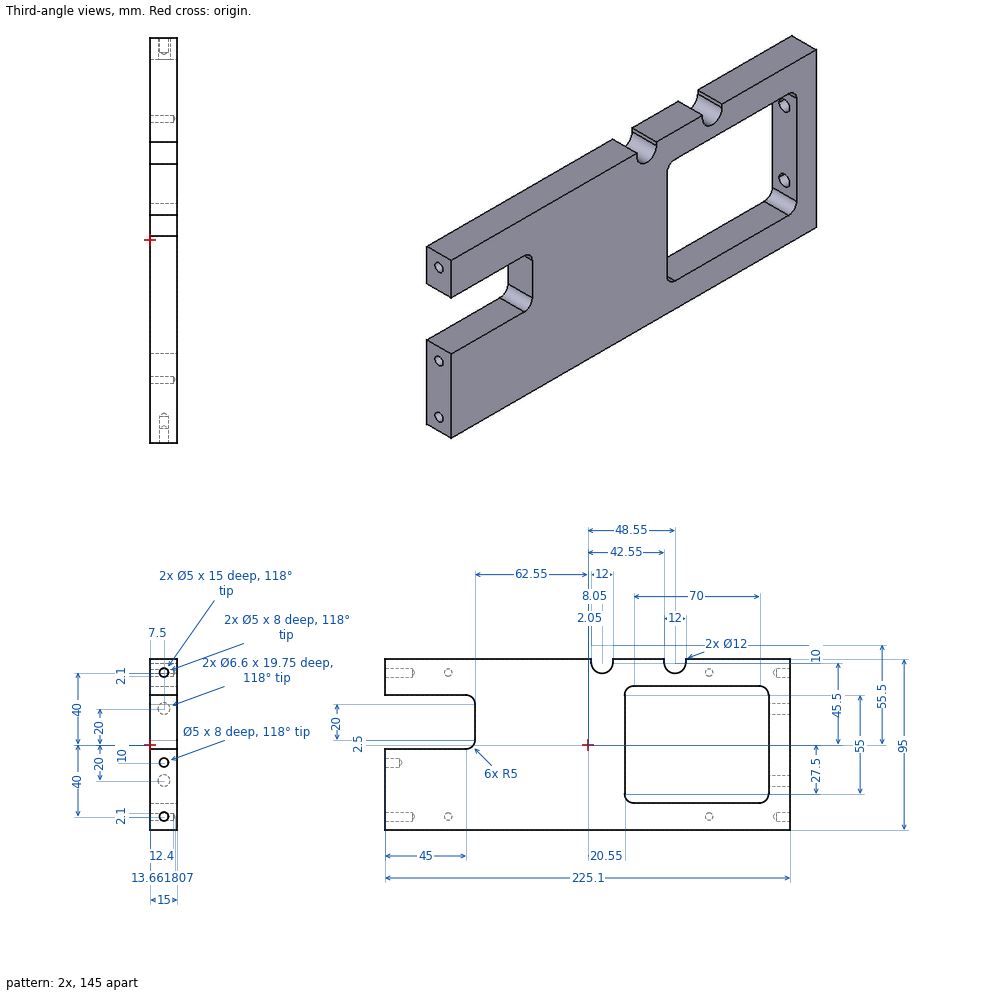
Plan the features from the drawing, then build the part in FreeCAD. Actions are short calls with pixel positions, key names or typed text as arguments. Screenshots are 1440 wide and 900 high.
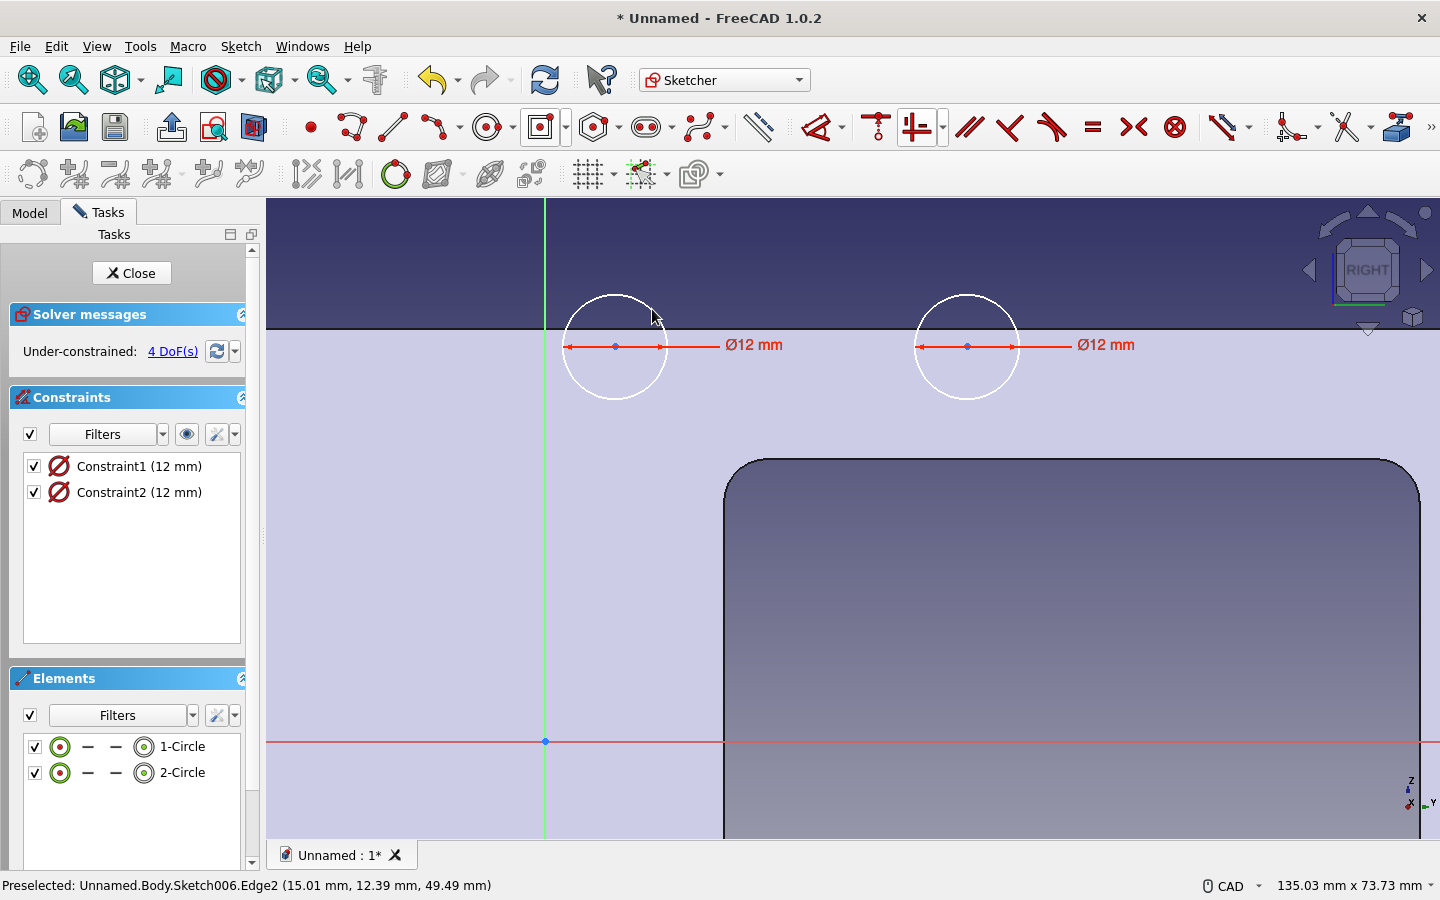
click(967, 347)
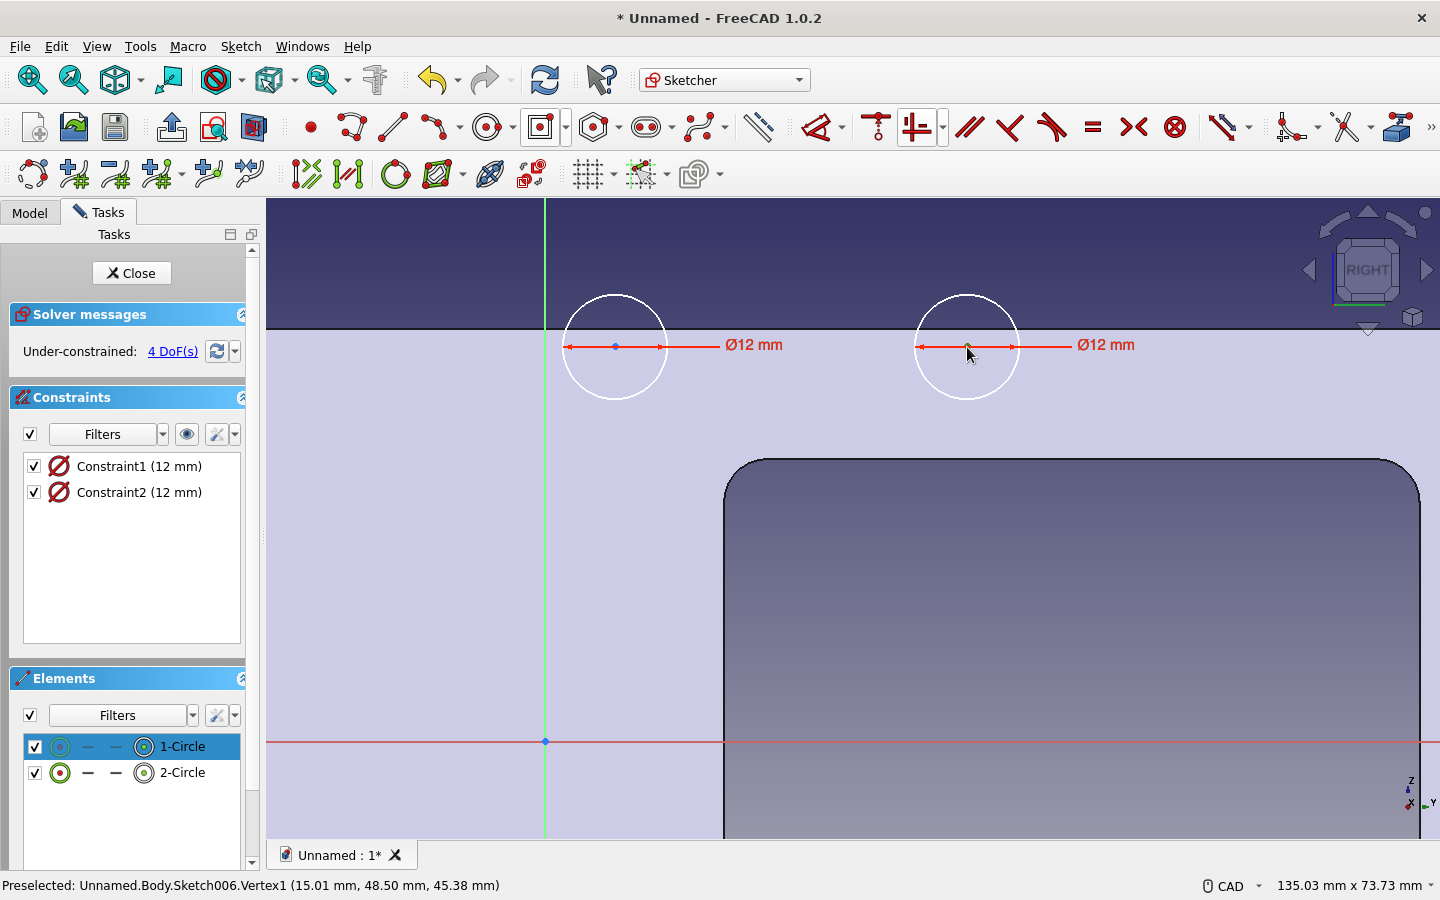
click(615, 347)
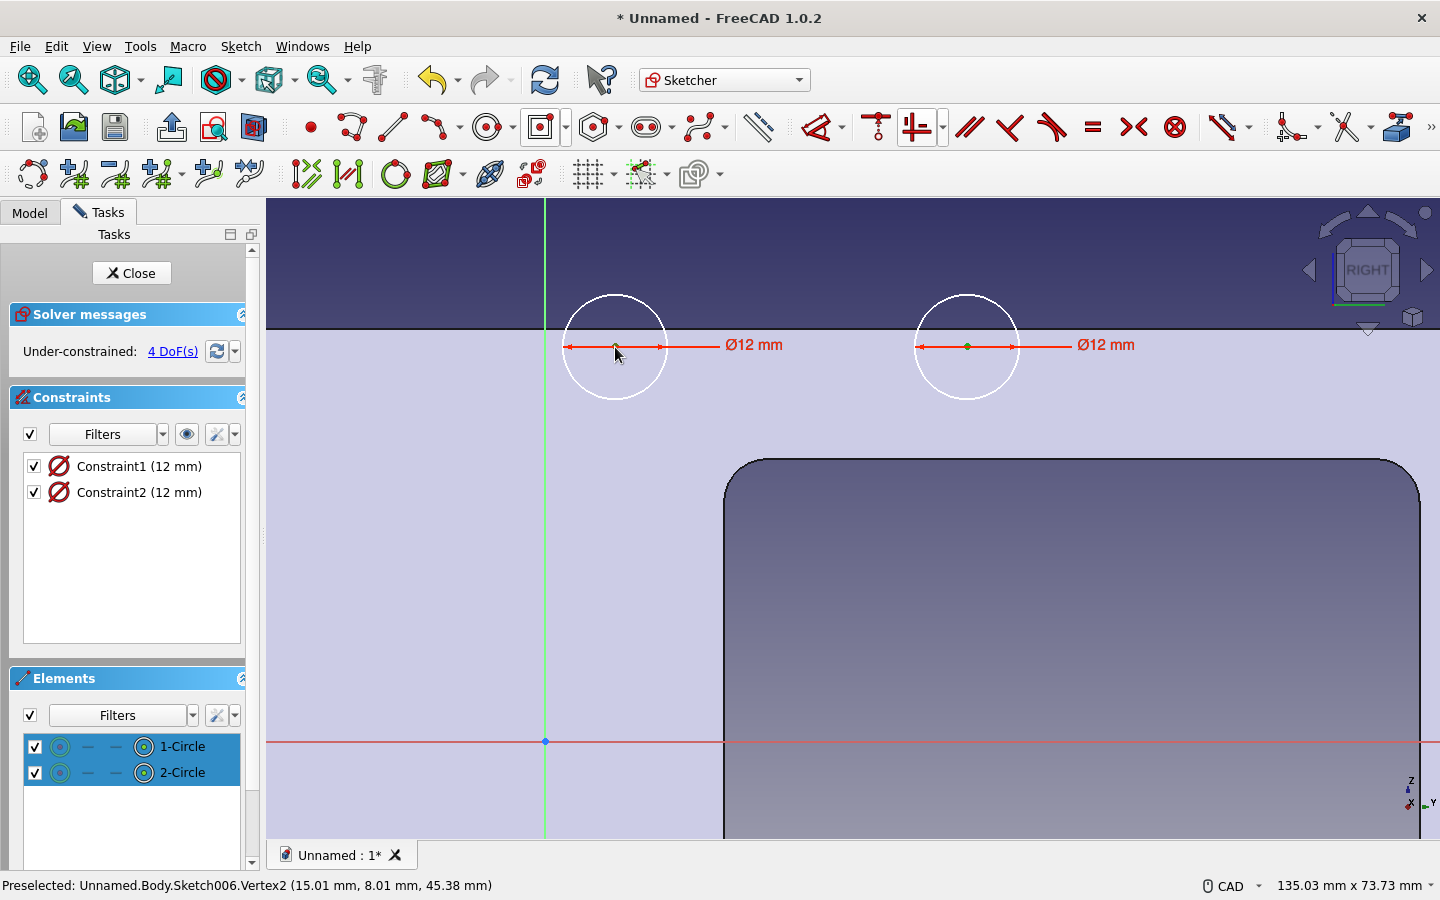
key(h)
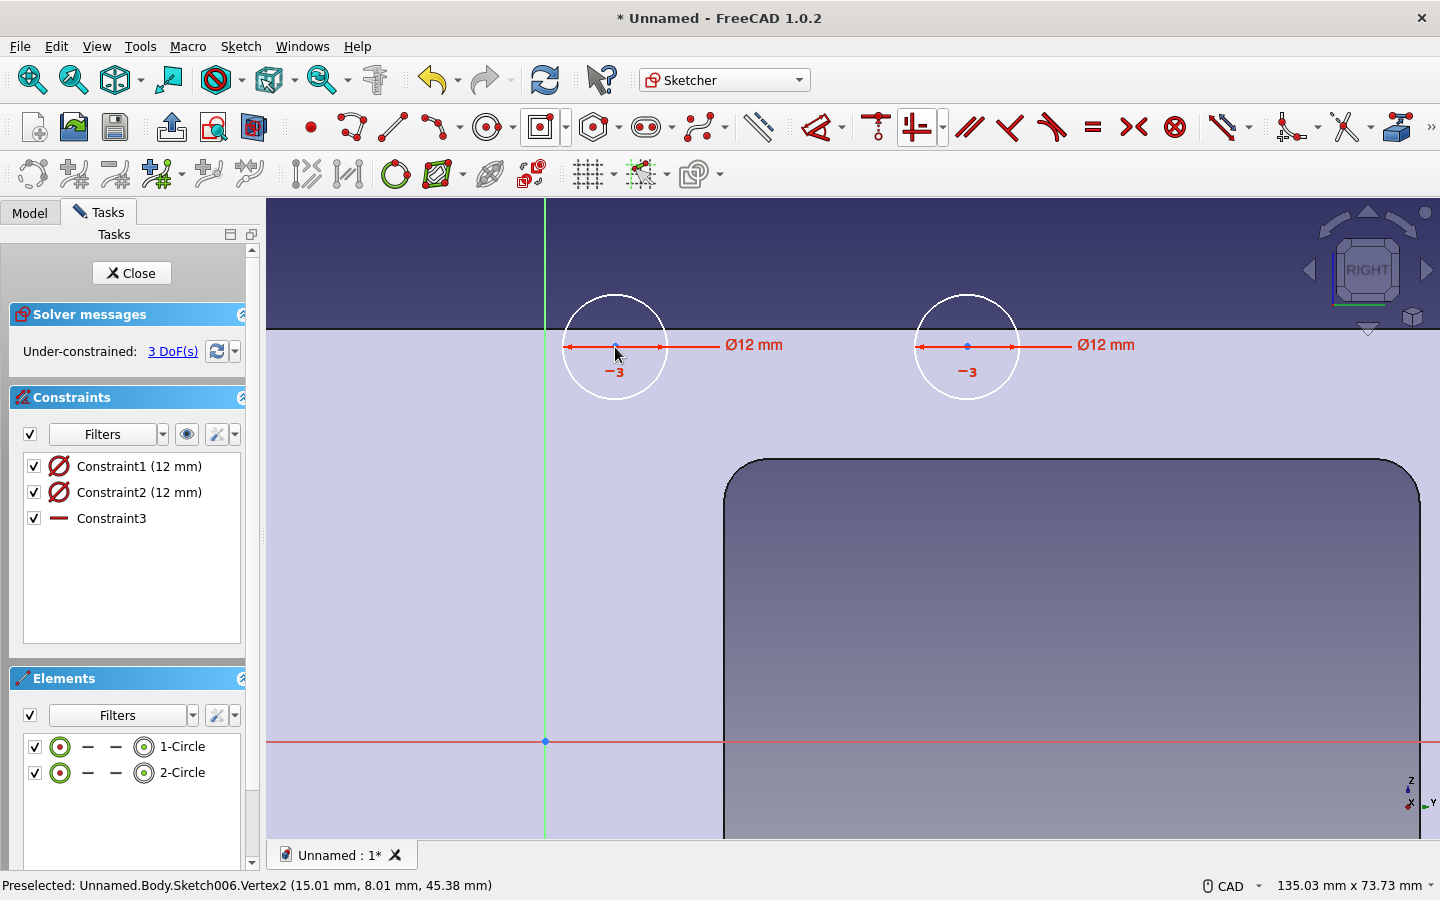
click(816, 128)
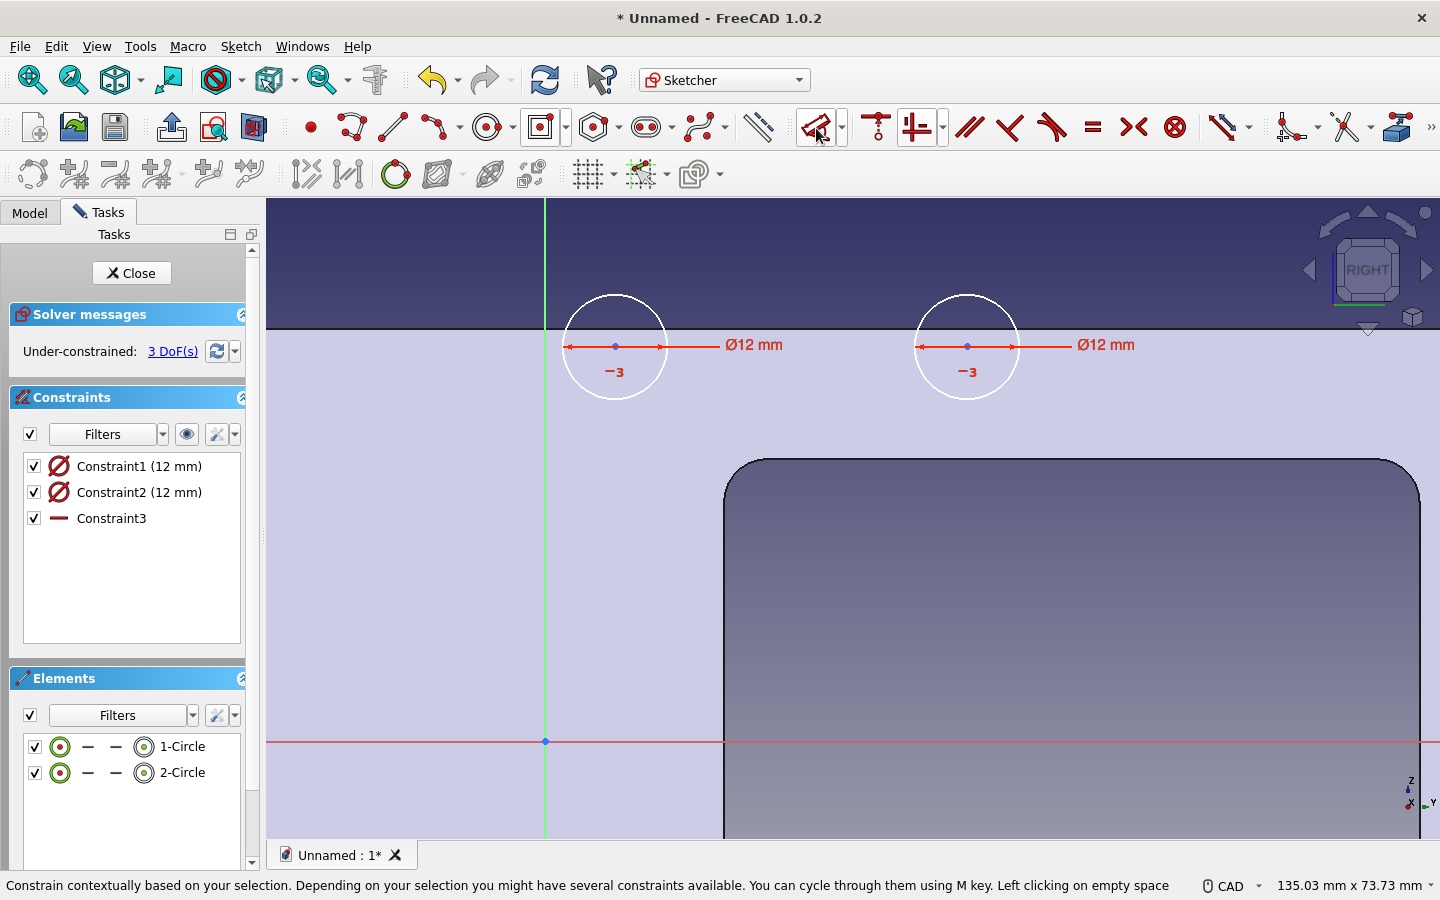
click(967, 347)
click(511, 544)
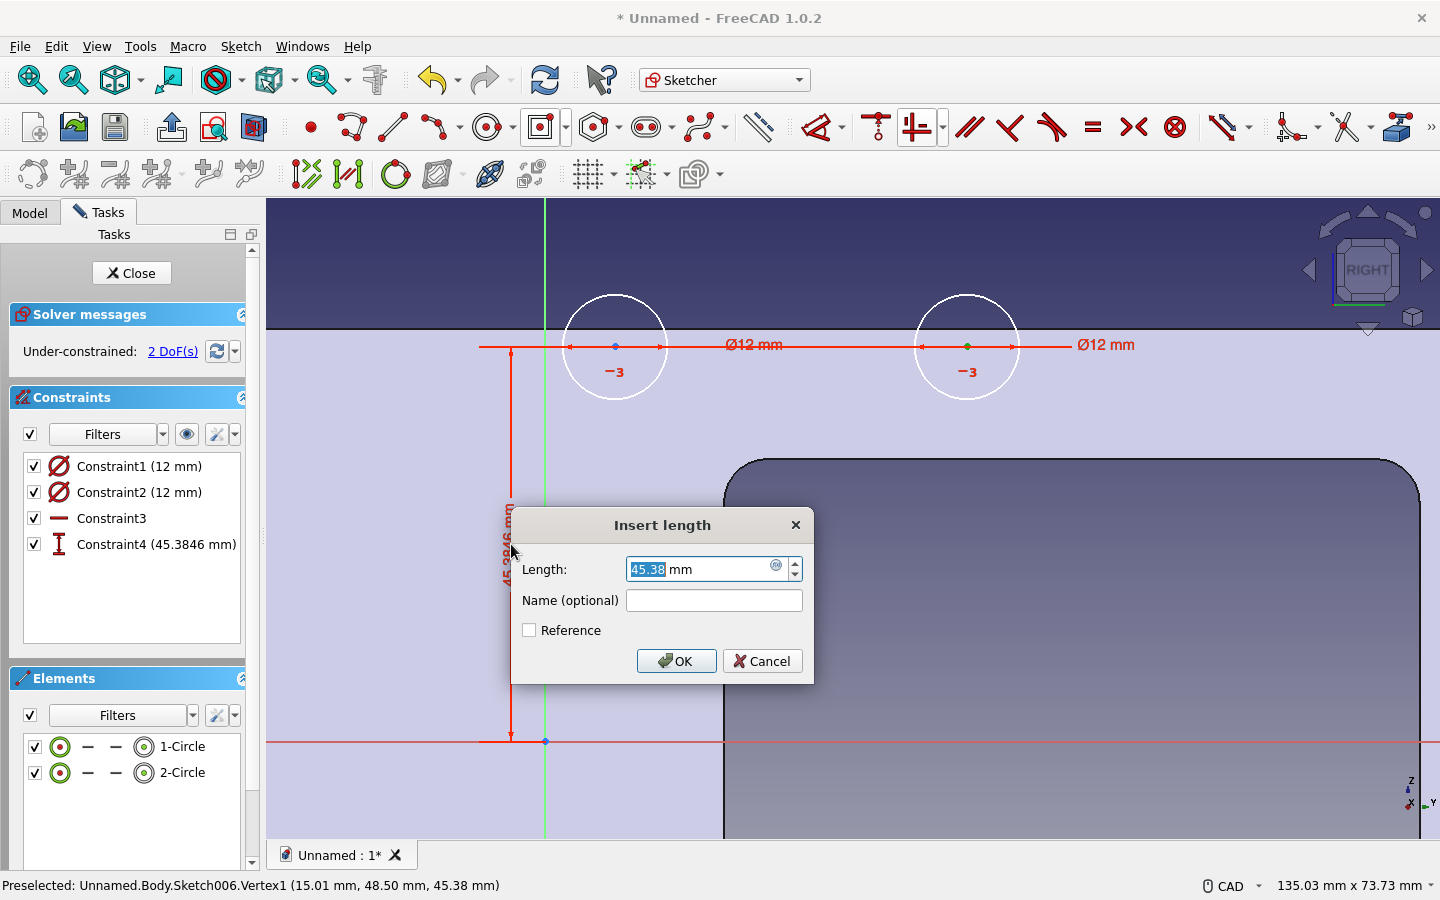
text(45.5)
key(Return)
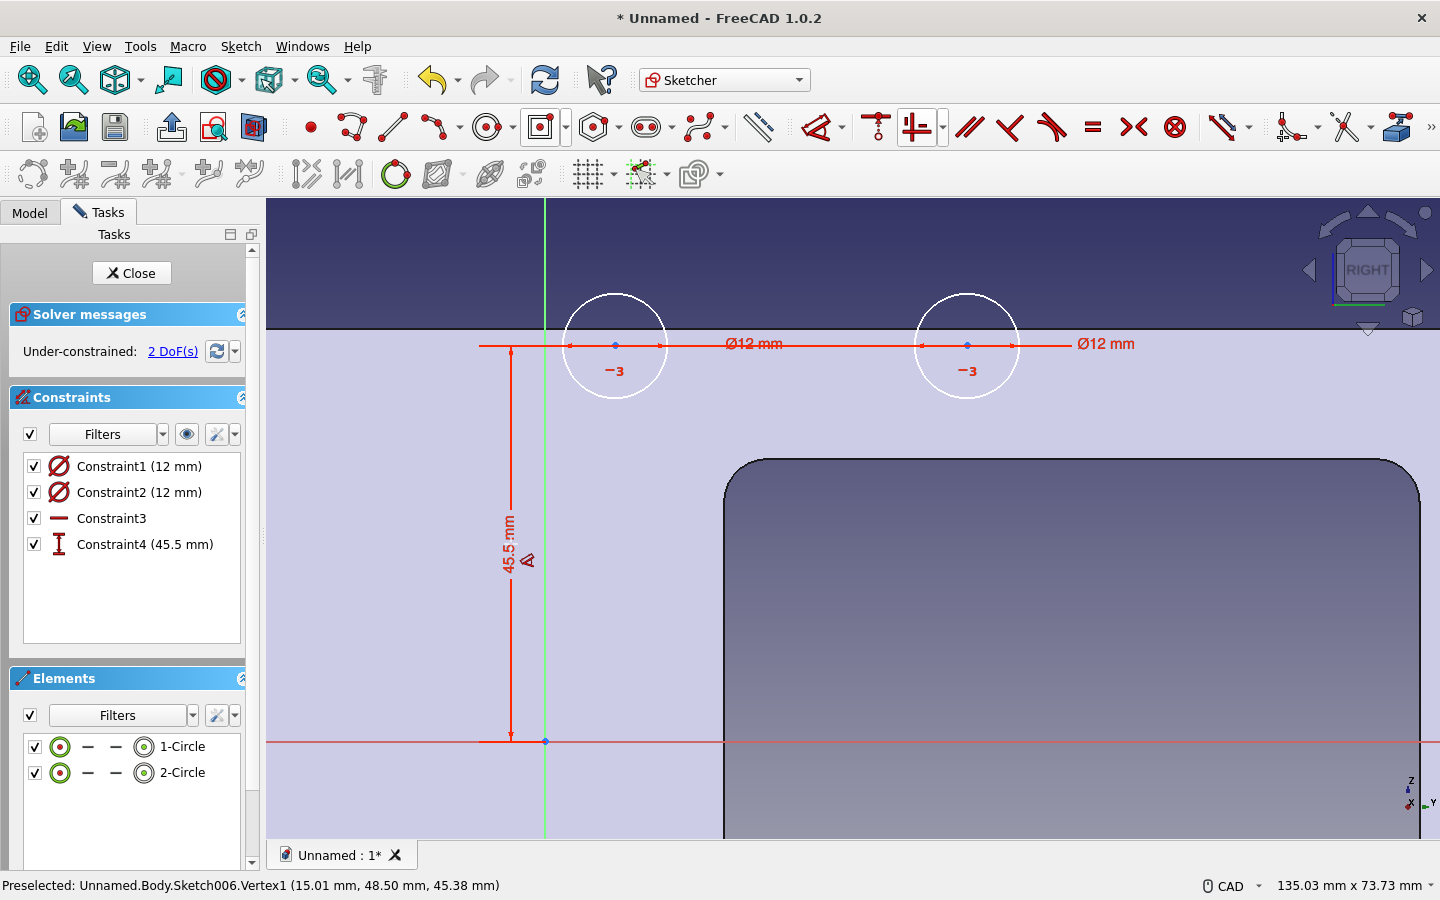
click(615, 346)
click(580, 776)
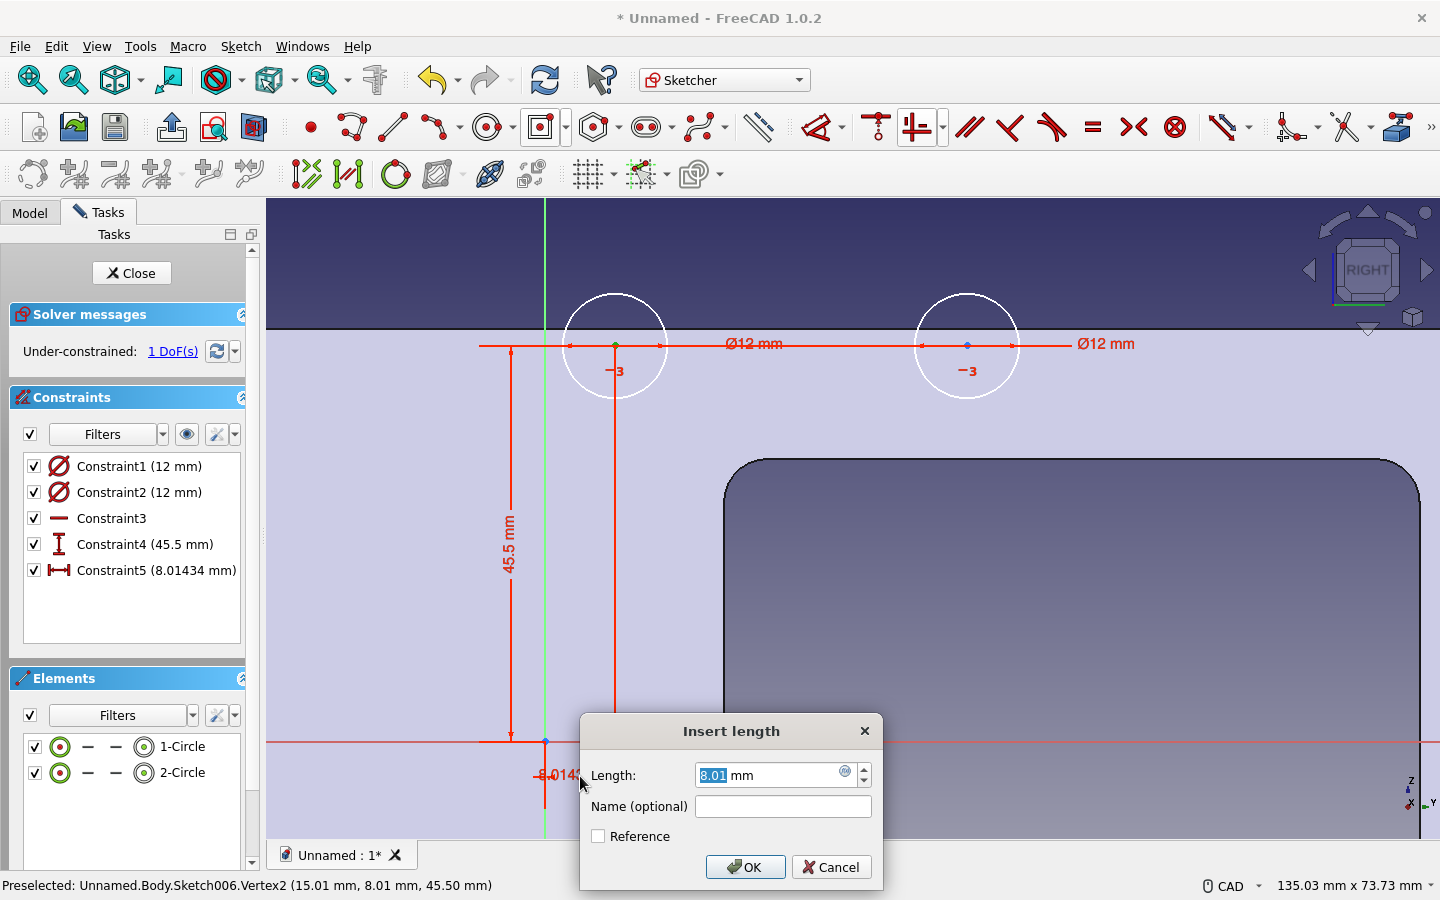
text(8.05)
key(Return)